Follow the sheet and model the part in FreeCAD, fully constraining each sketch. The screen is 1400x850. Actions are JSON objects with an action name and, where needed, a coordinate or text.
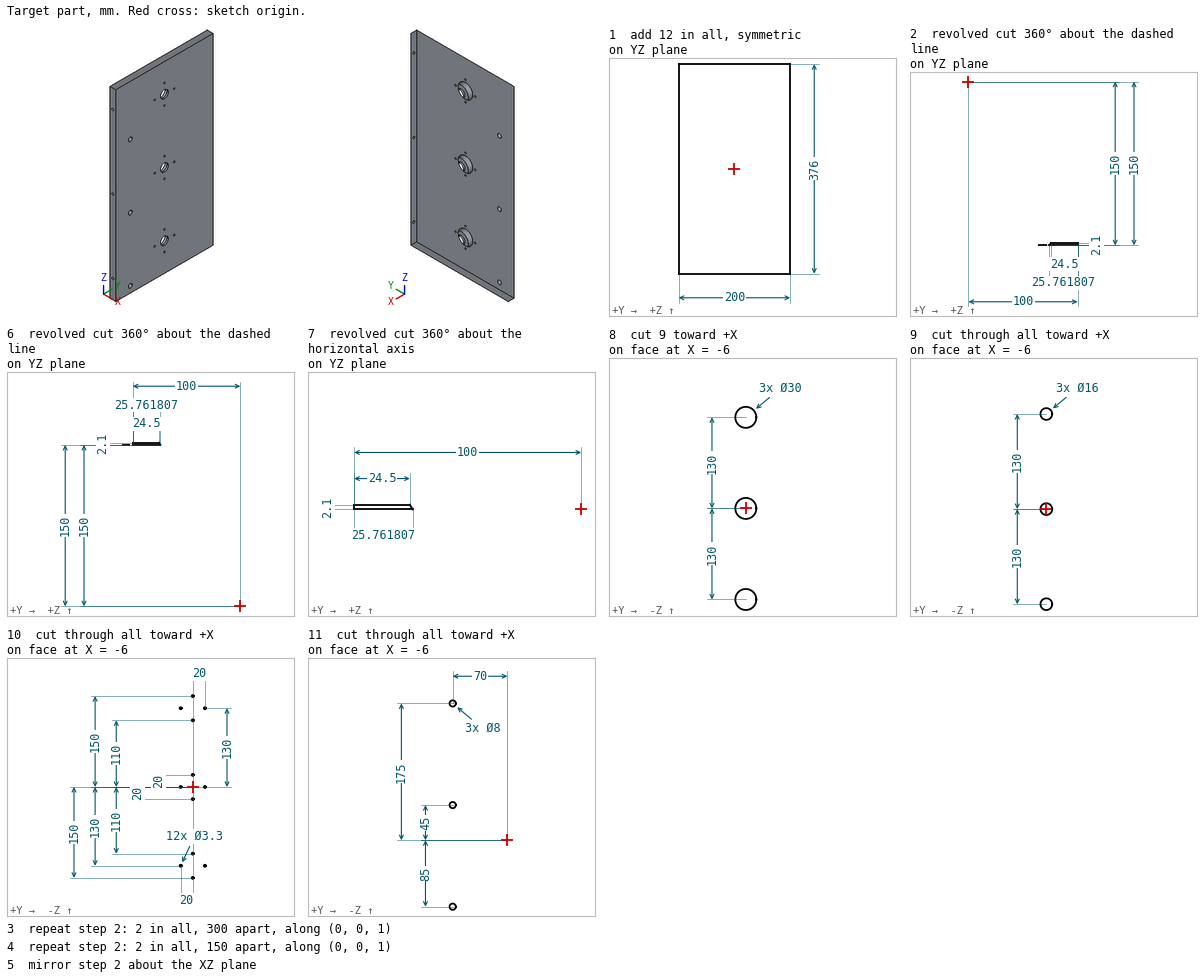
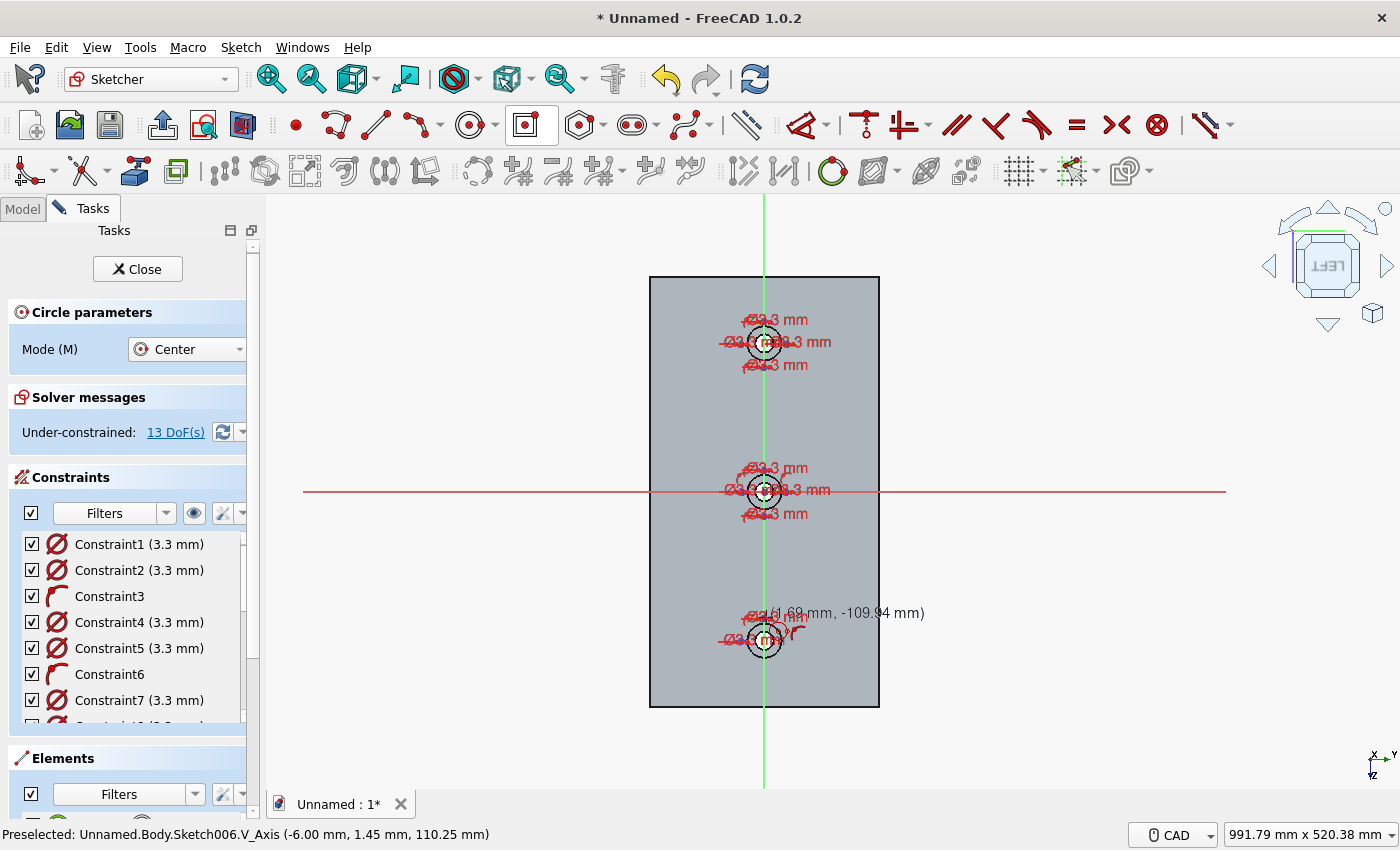
{"action": "scroll", "coordinate": [787, 641], "scroll_direction": "up", "scroll_amount": 13}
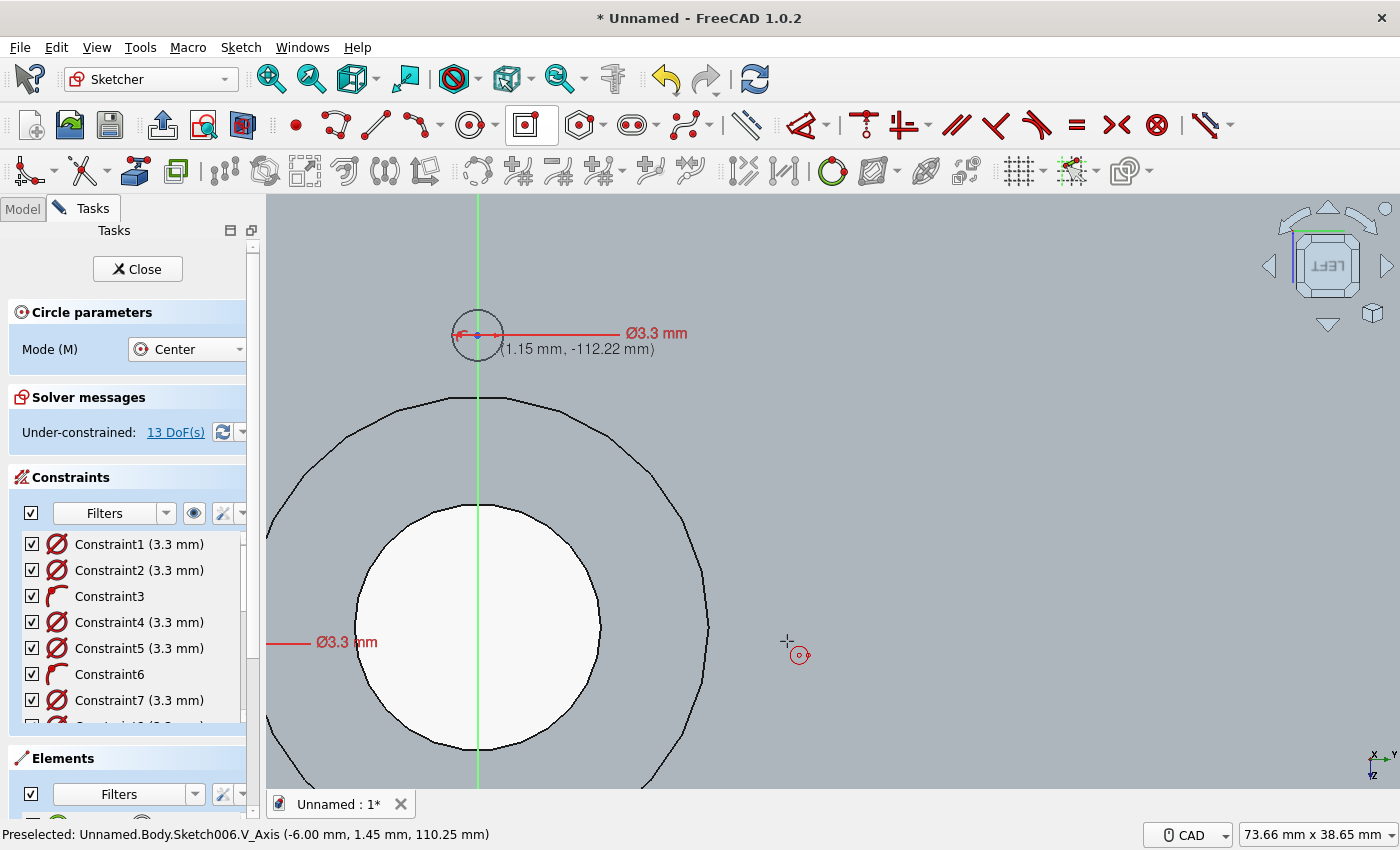
{"action": "scroll", "coordinate": [788, 641], "scroll_direction": "down", "scroll_amount": 13}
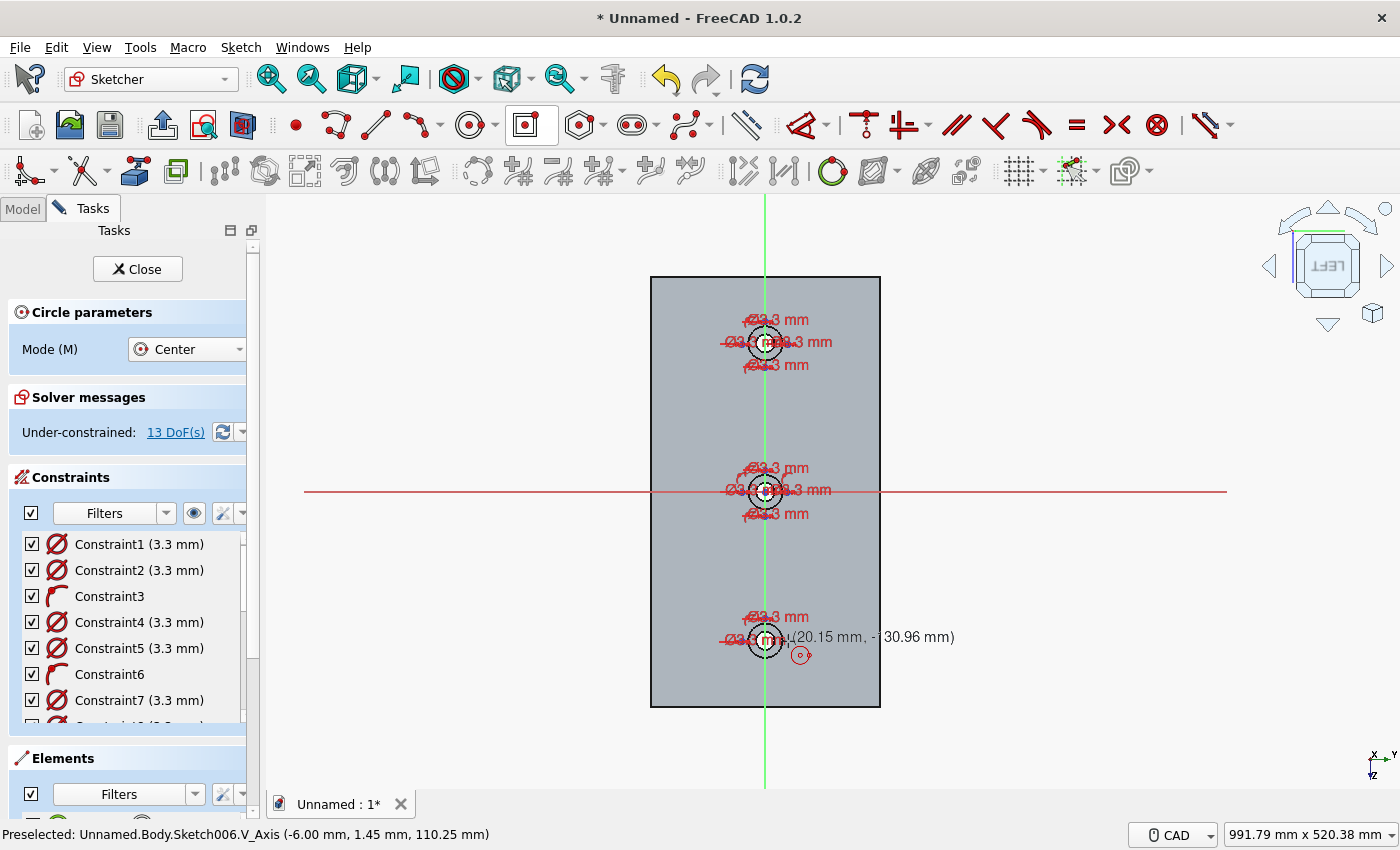
{"action": "left_click", "coordinate": [788, 641]}
{"action": "mouse_move", "coordinate": [790, 639]}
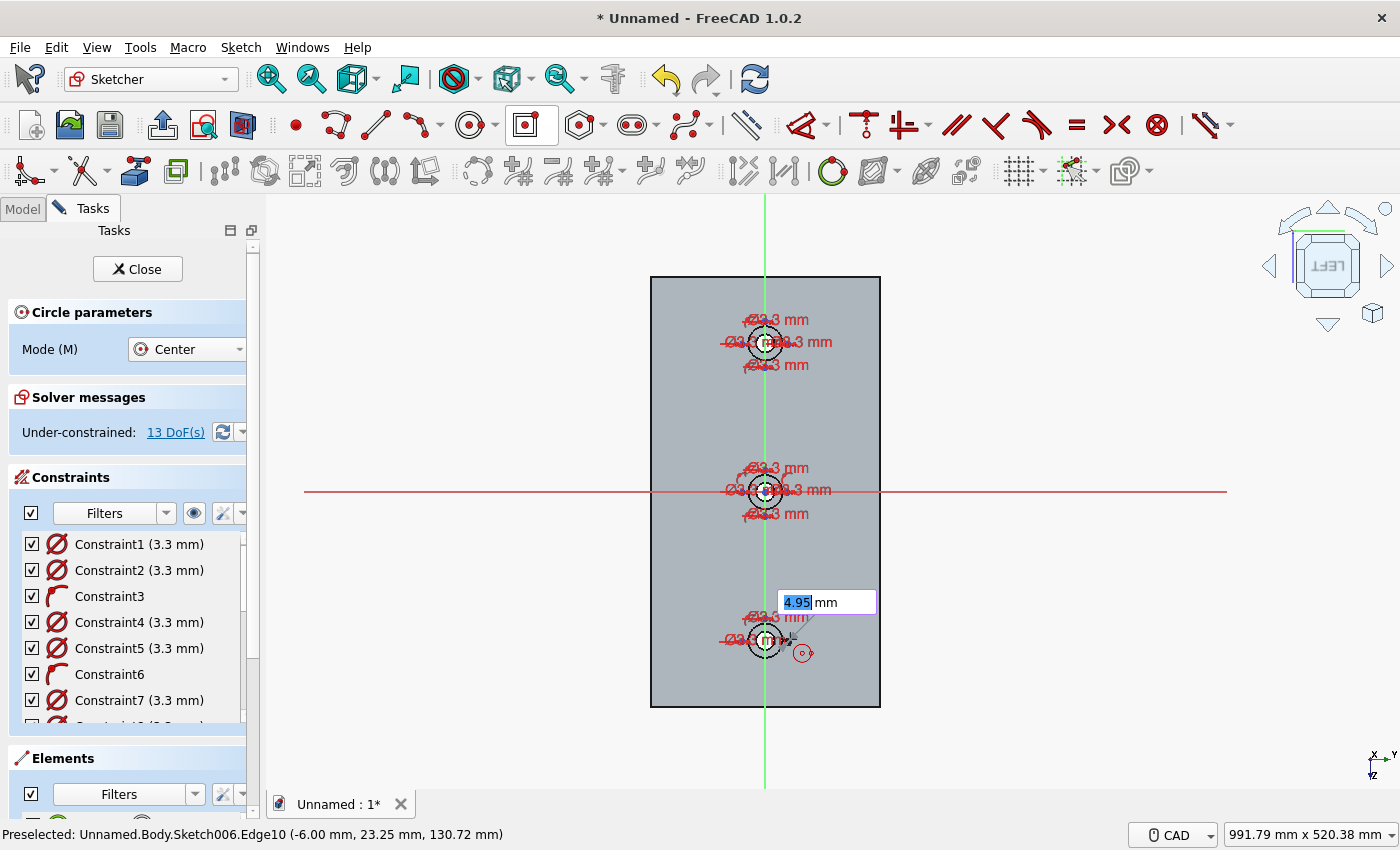
{"action": "type", "text": "3.3"}
{"action": "key", "text": "Return"}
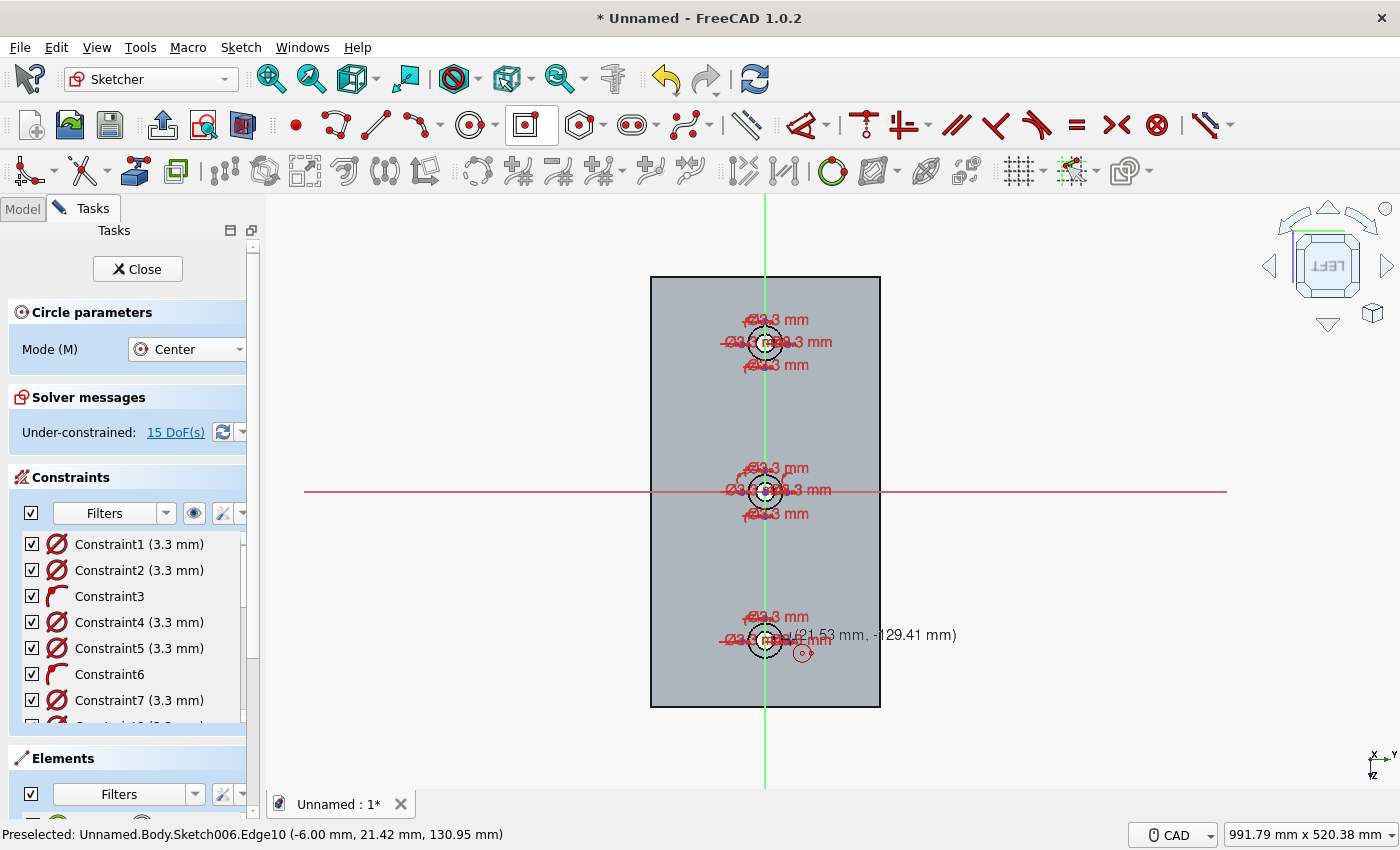
{"action": "scroll", "coordinate": [765, 664], "scroll_direction": "up", "scroll_amount": 13}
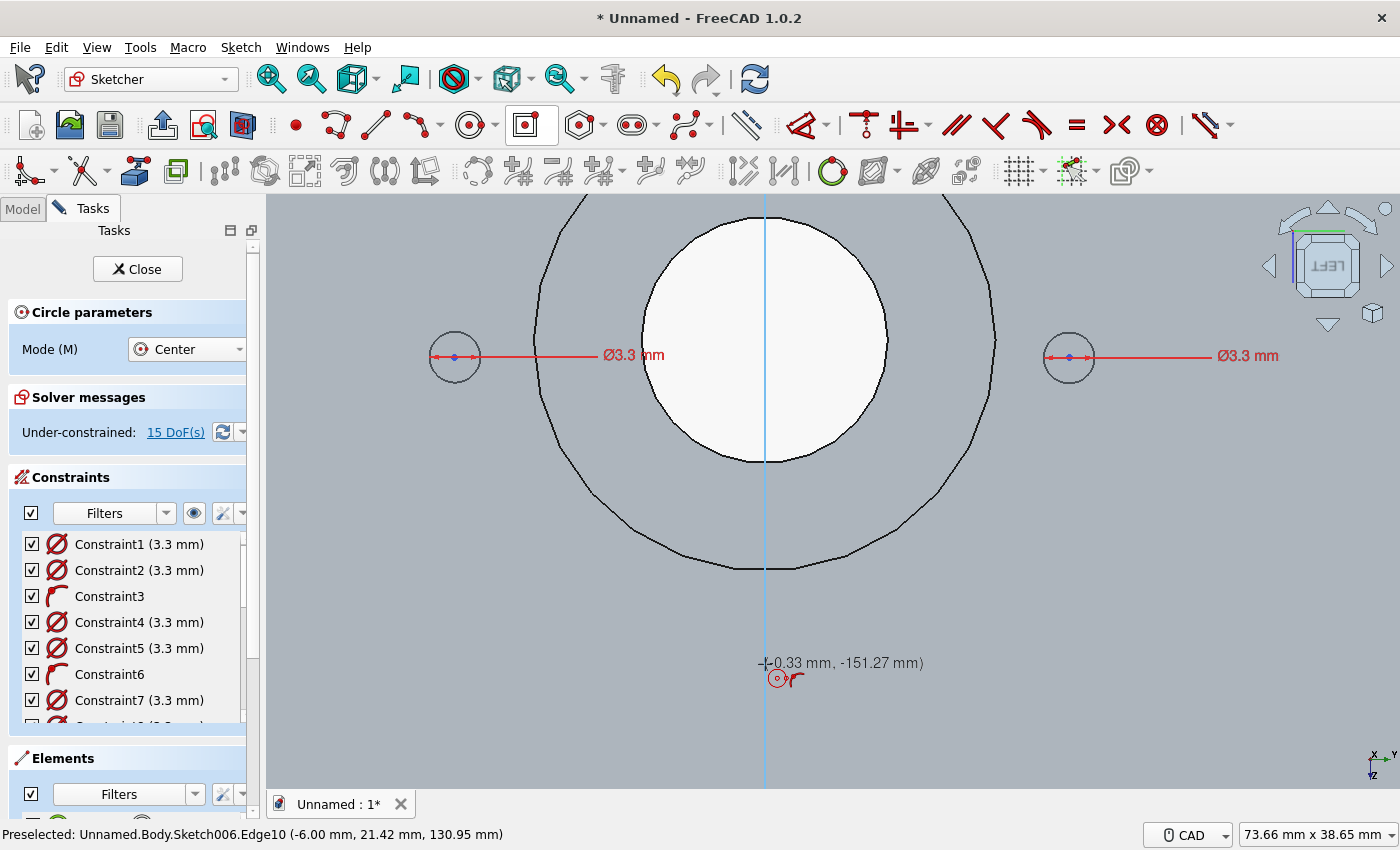
{"action": "scroll", "coordinate": [764, 664], "scroll_direction": "down", "scroll_amount": 13}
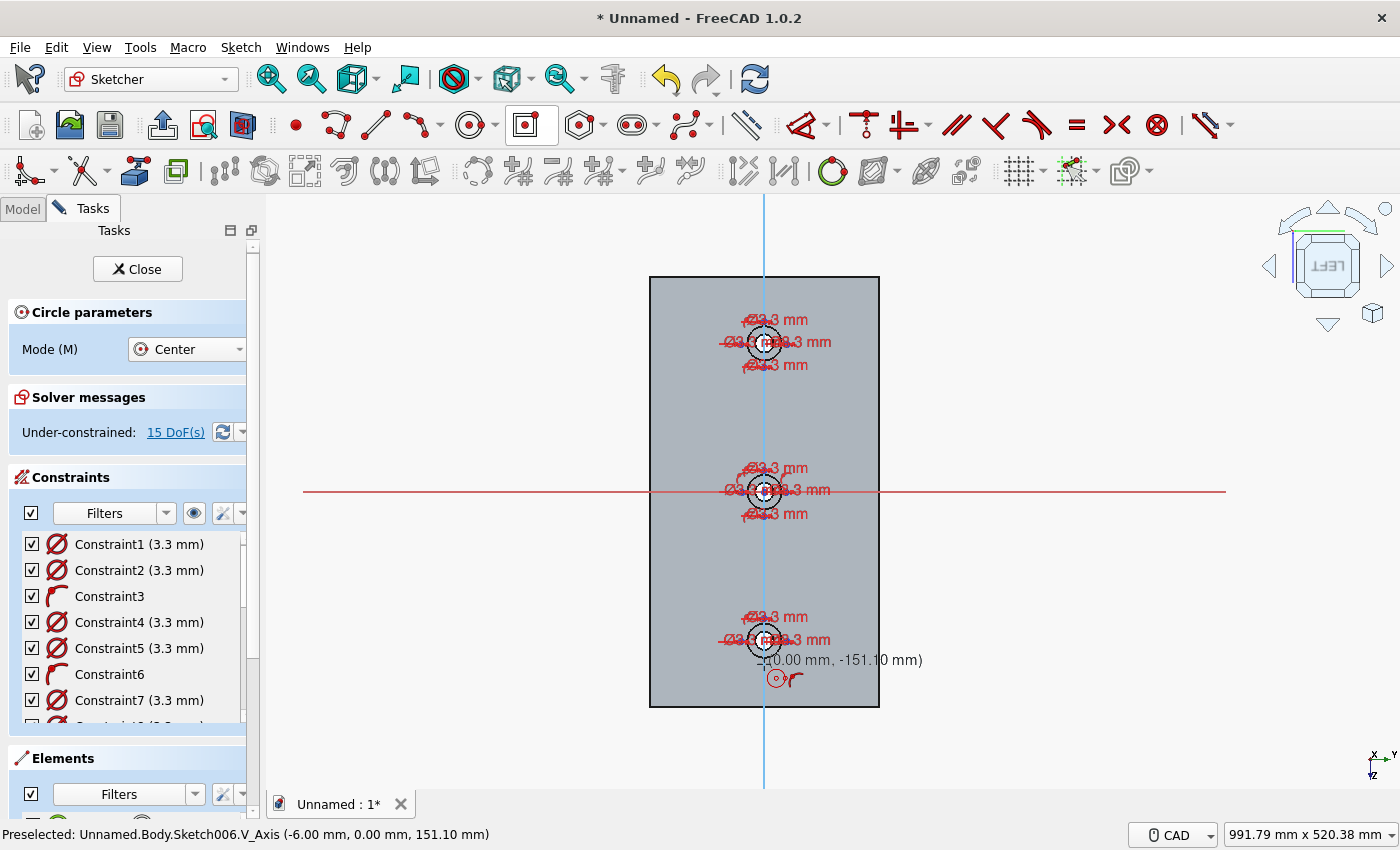
{"action": "left_click", "coordinate": [764, 664]}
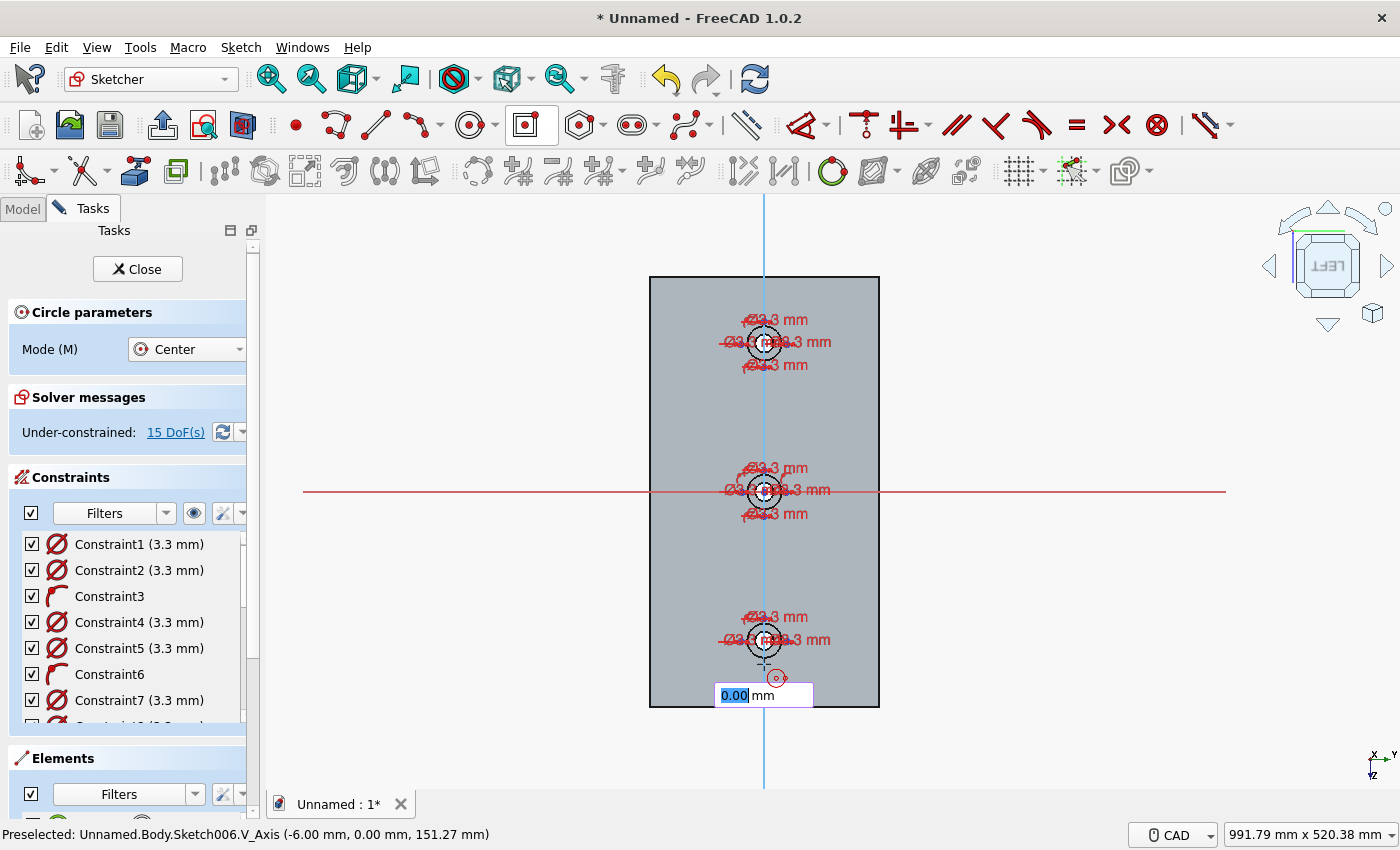
{"action": "scroll", "coordinate": [766, 663], "scroll_direction": "up", "scroll_amount": 11}
{"action": "mouse_move", "coordinate": [765, 656]}